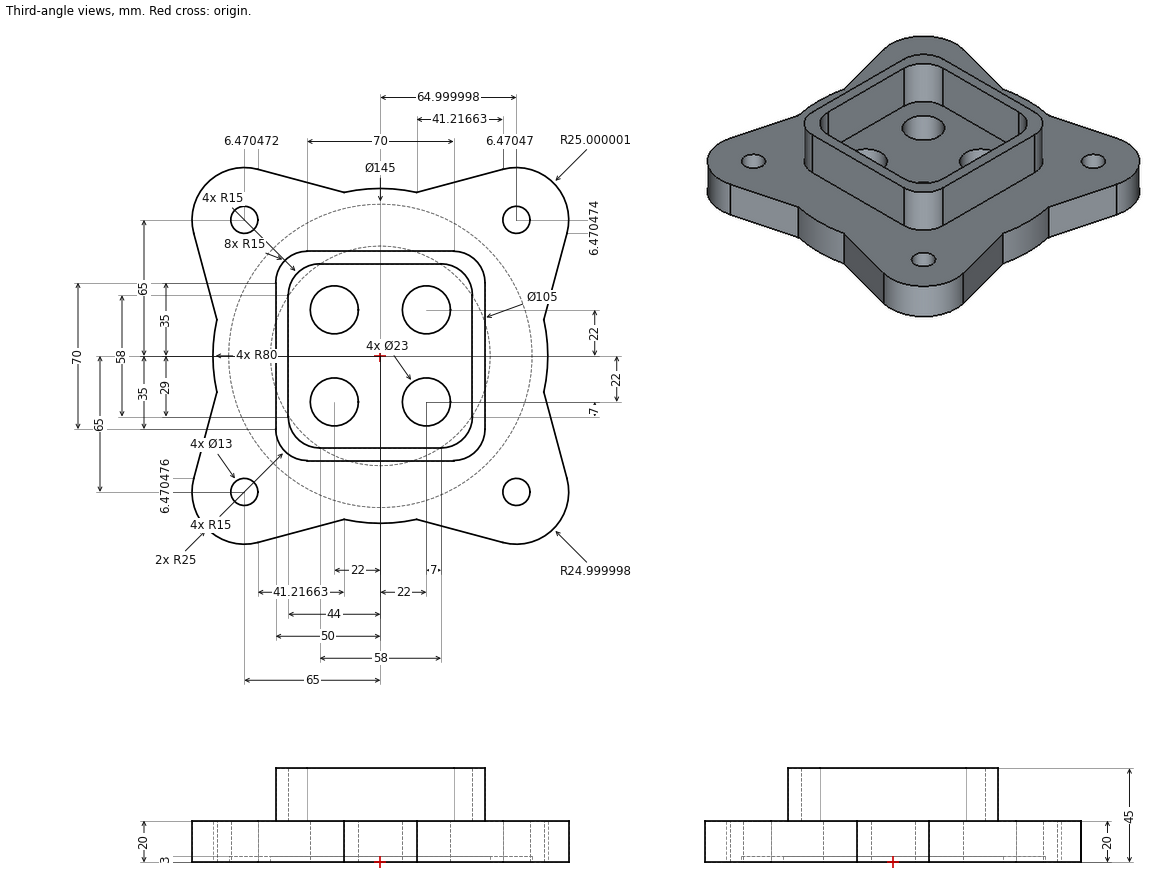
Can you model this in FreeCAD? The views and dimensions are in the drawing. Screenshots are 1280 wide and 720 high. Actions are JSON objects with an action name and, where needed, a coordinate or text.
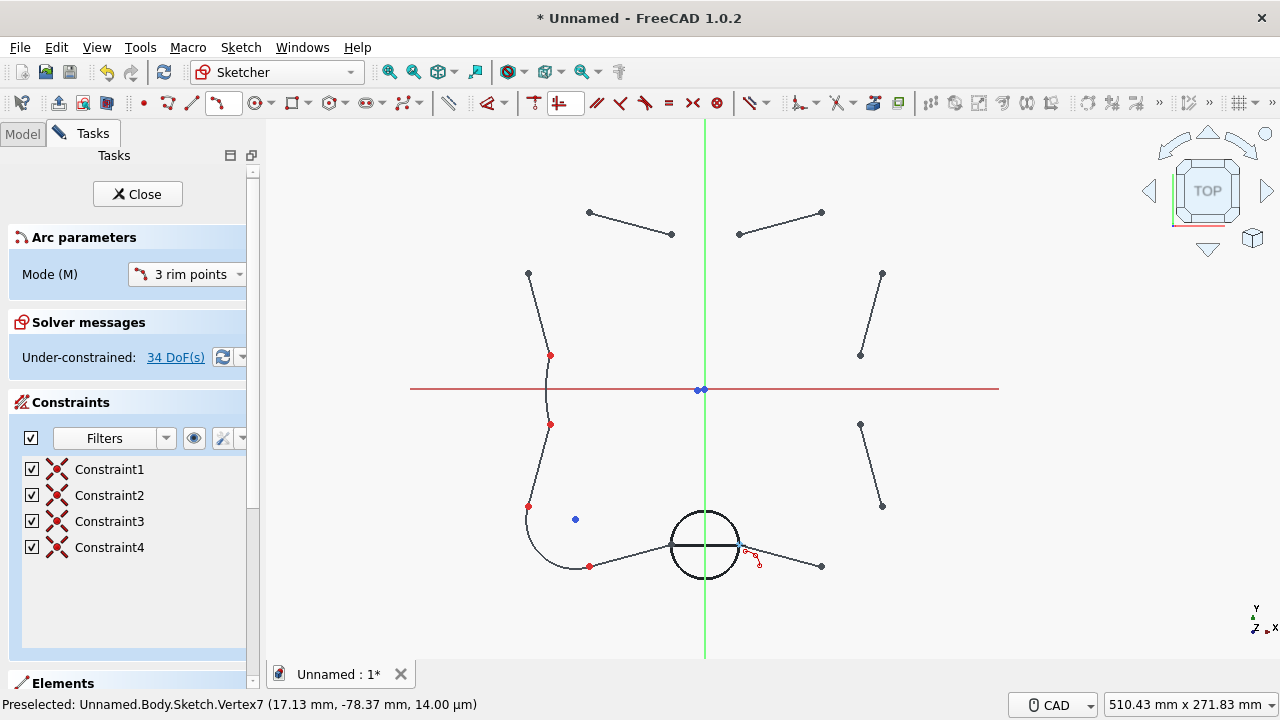
{"action": "scroll", "coordinate": [705, 548], "scroll_direction": "up", "scroll_amount": 8}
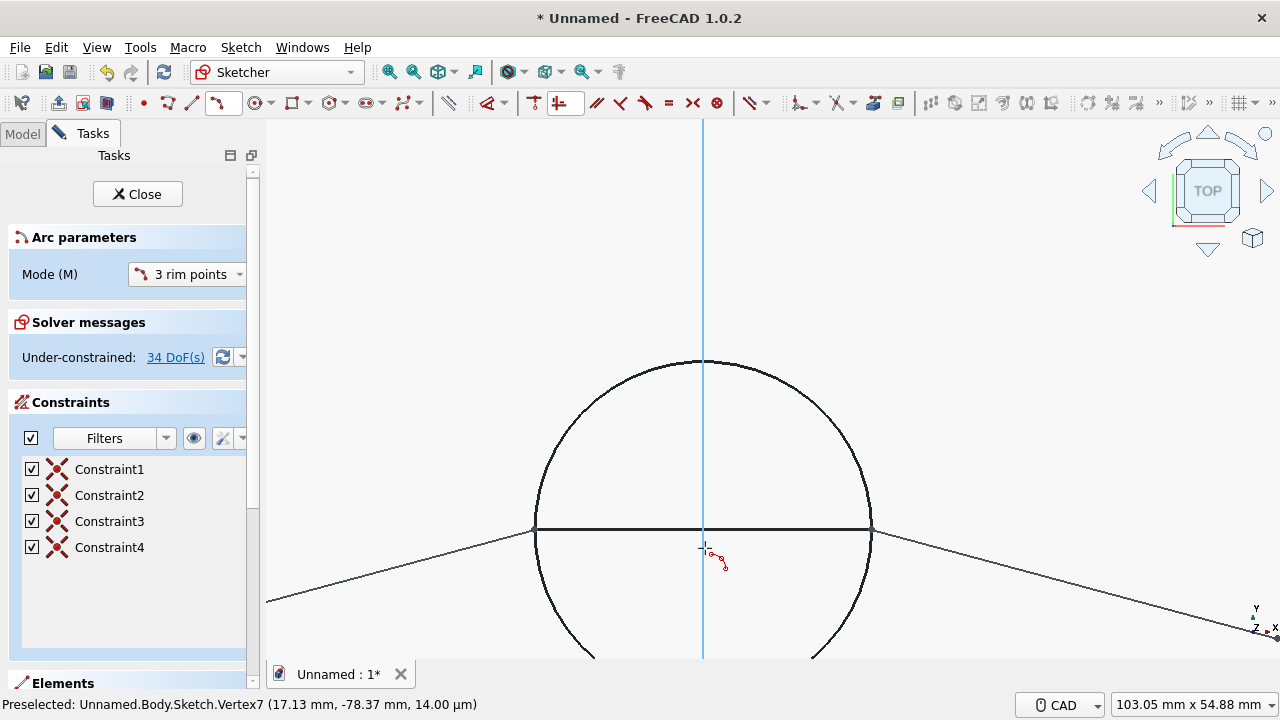
{"action": "left_click", "coordinate": [703, 546]}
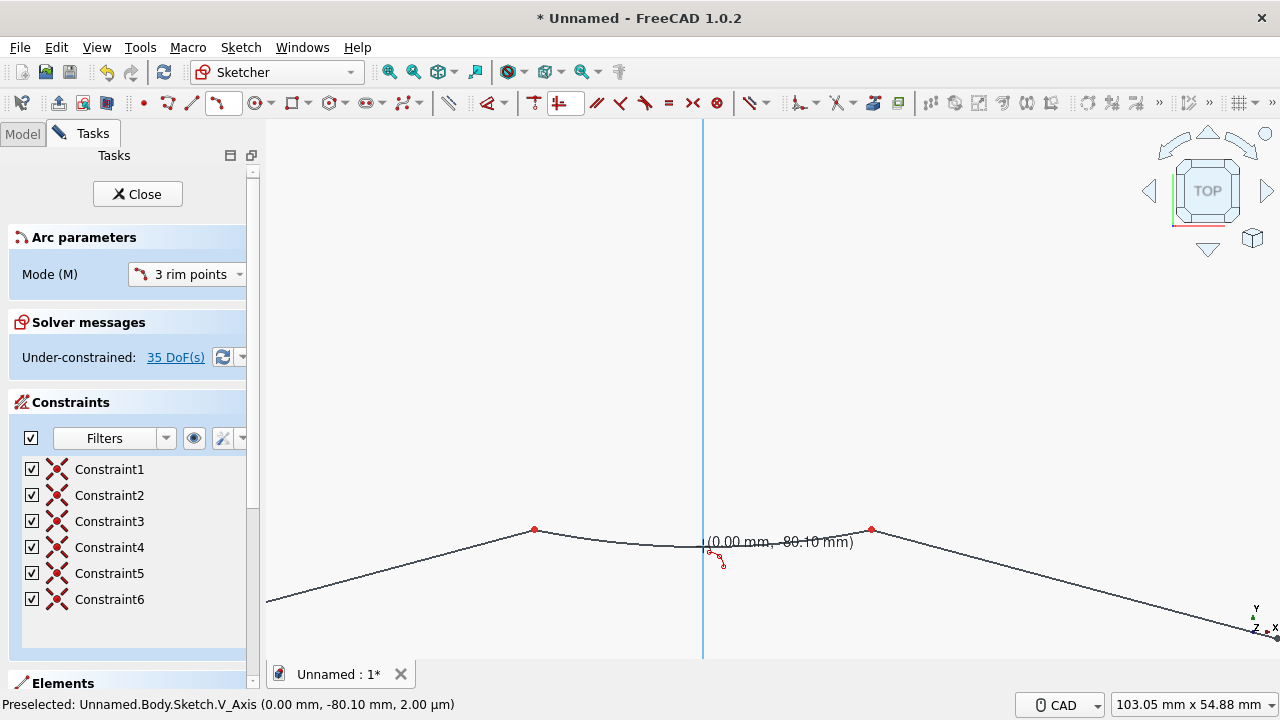
{"action": "scroll", "coordinate": [705, 548], "scroll_direction": "down", "scroll_amount": 8}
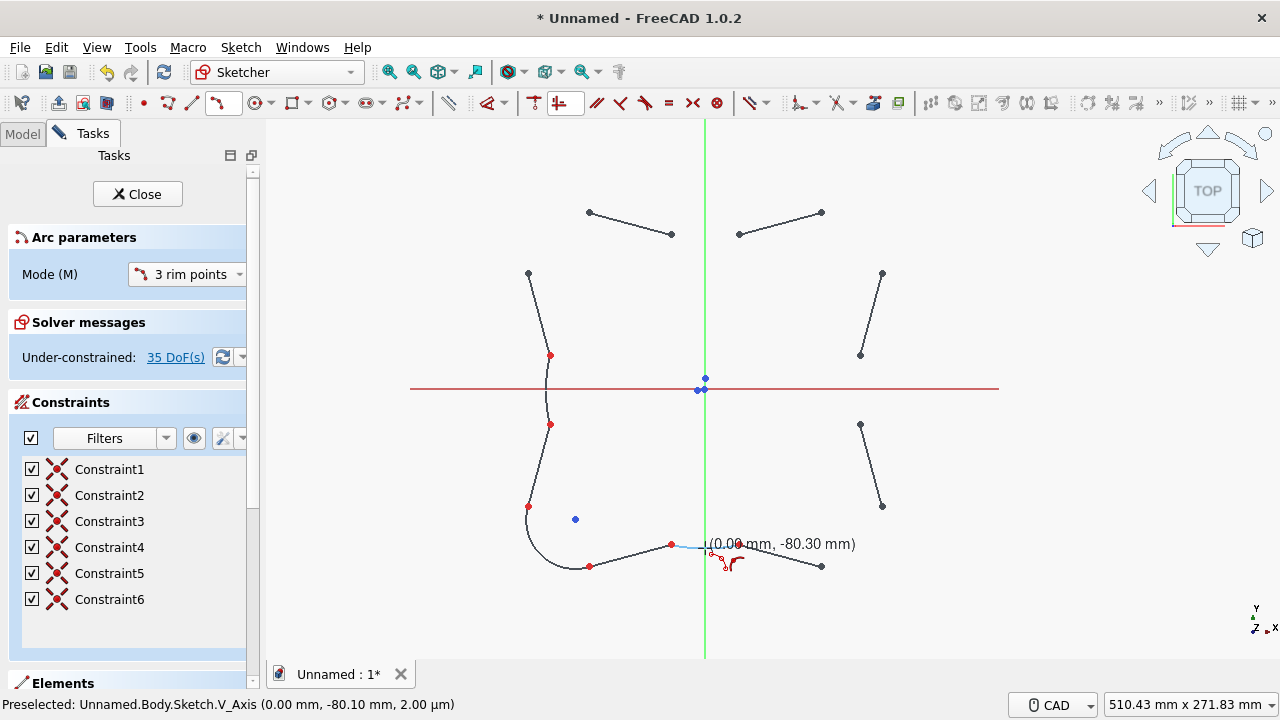
{"action": "left_click", "coordinate": [821, 567]}
{"action": "left_click", "coordinate": [882, 507]}
{"action": "left_click", "coordinate": [869, 554]}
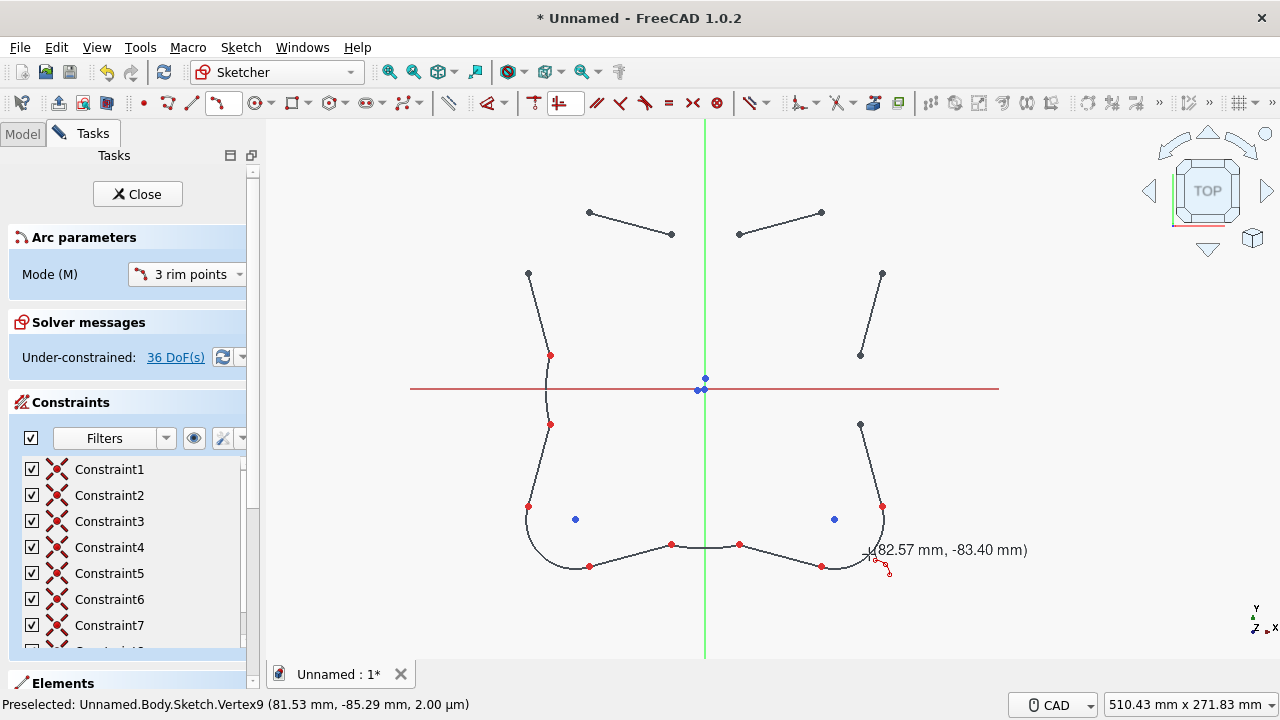
{"action": "left_click", "coordinate": [860, 425]}
{"action": "left_click", "coordinate": [860, 356]}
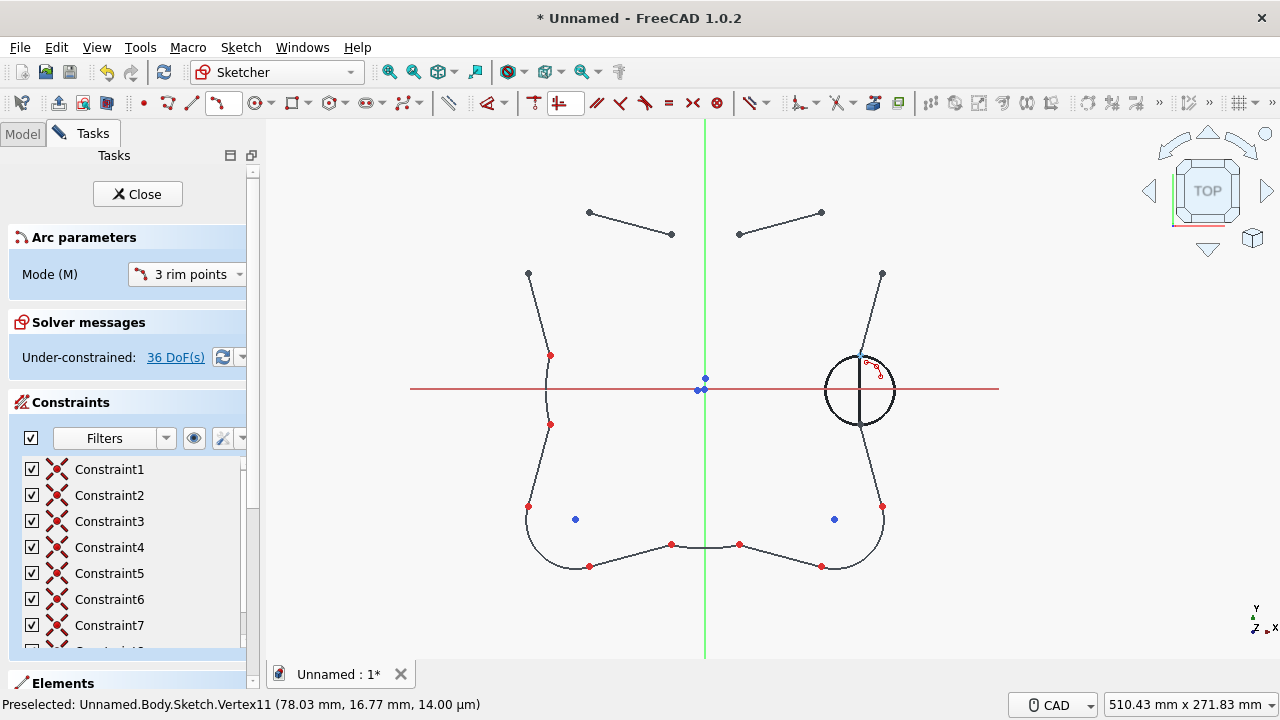
{"action": "scroll", "coordinate": [864, 396], "scroll_direction": "up", "scroll_amount": 8}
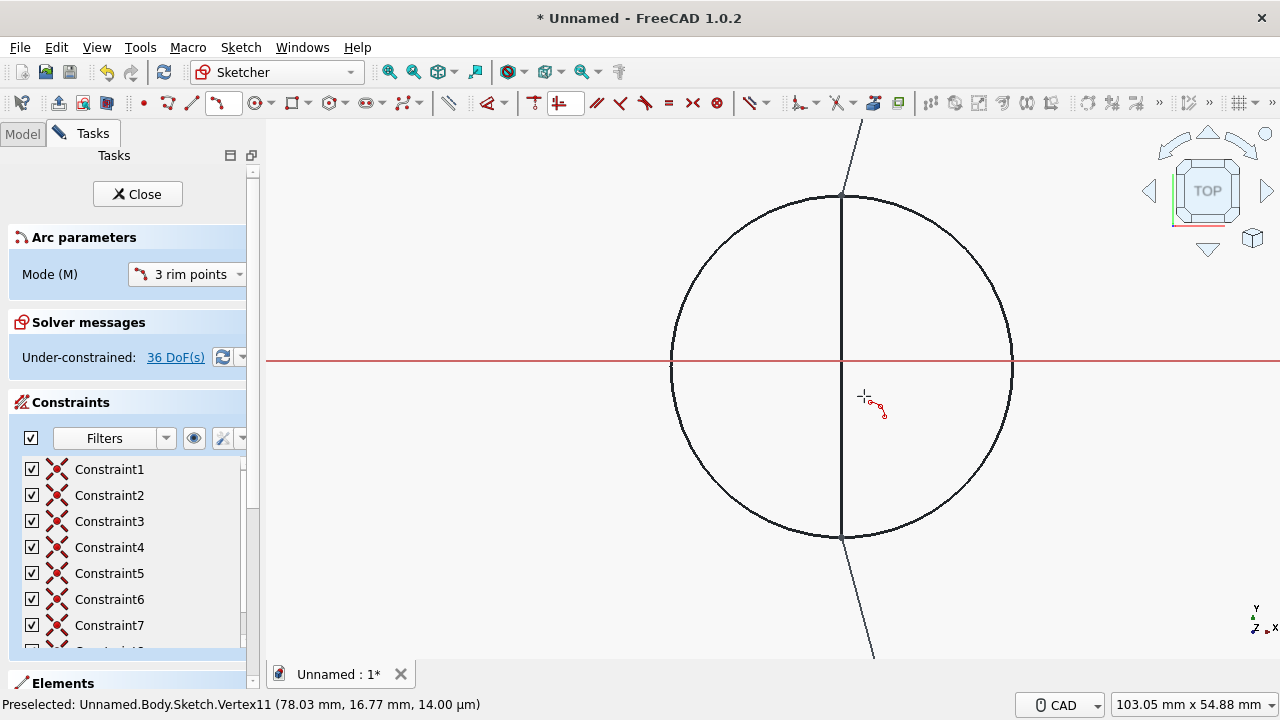
{"action": "left_click", "coordinate": [860, 395]}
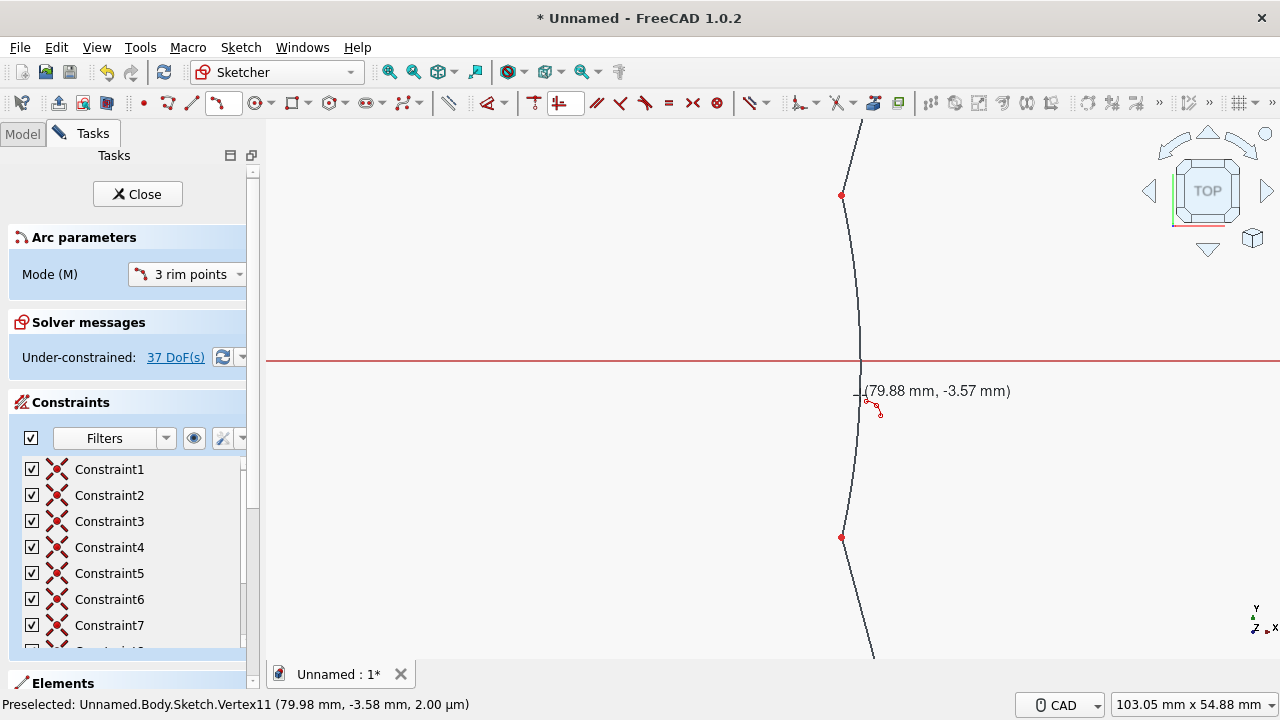
{"action": "scroll", "coordinate": [864, 396], "scroll_direction": "down", "scroll_amount": 8}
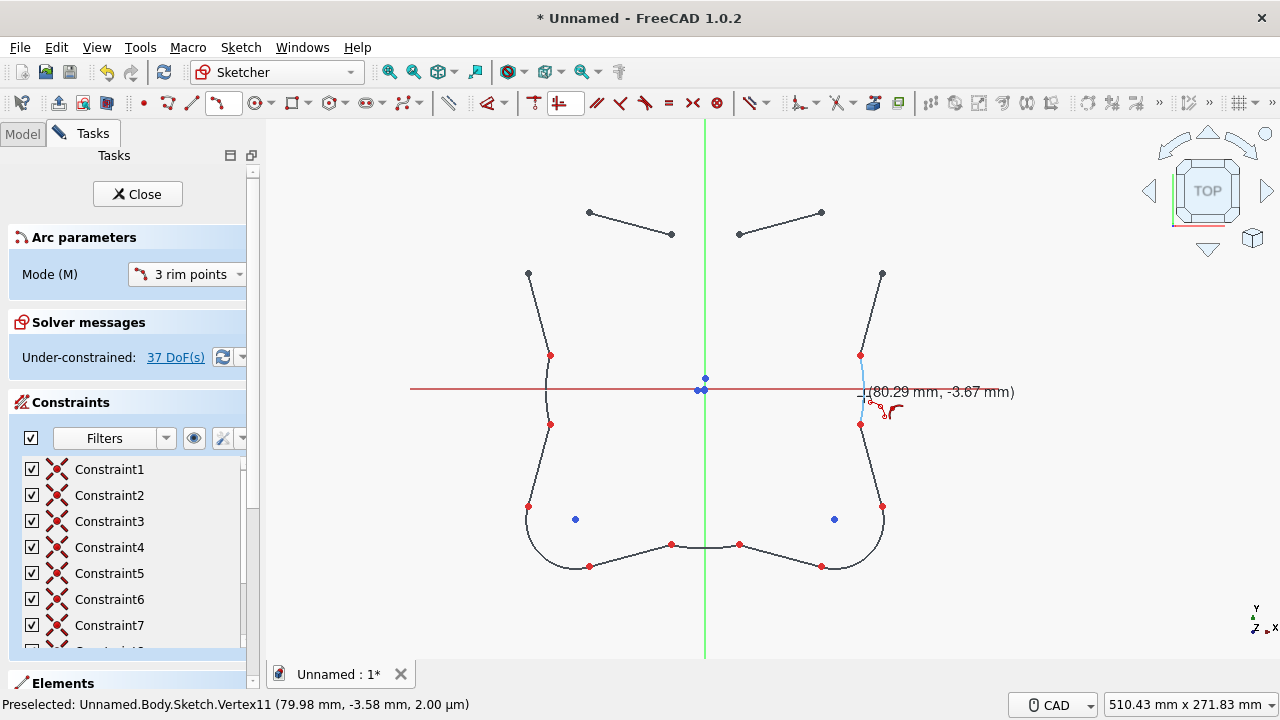
{"action": "left_click", "coordinate": [882, 274]}
{"action": "left_click", "coordinate": [821, 213]}
{"action": "left_click", "coordinate": [869, 225]}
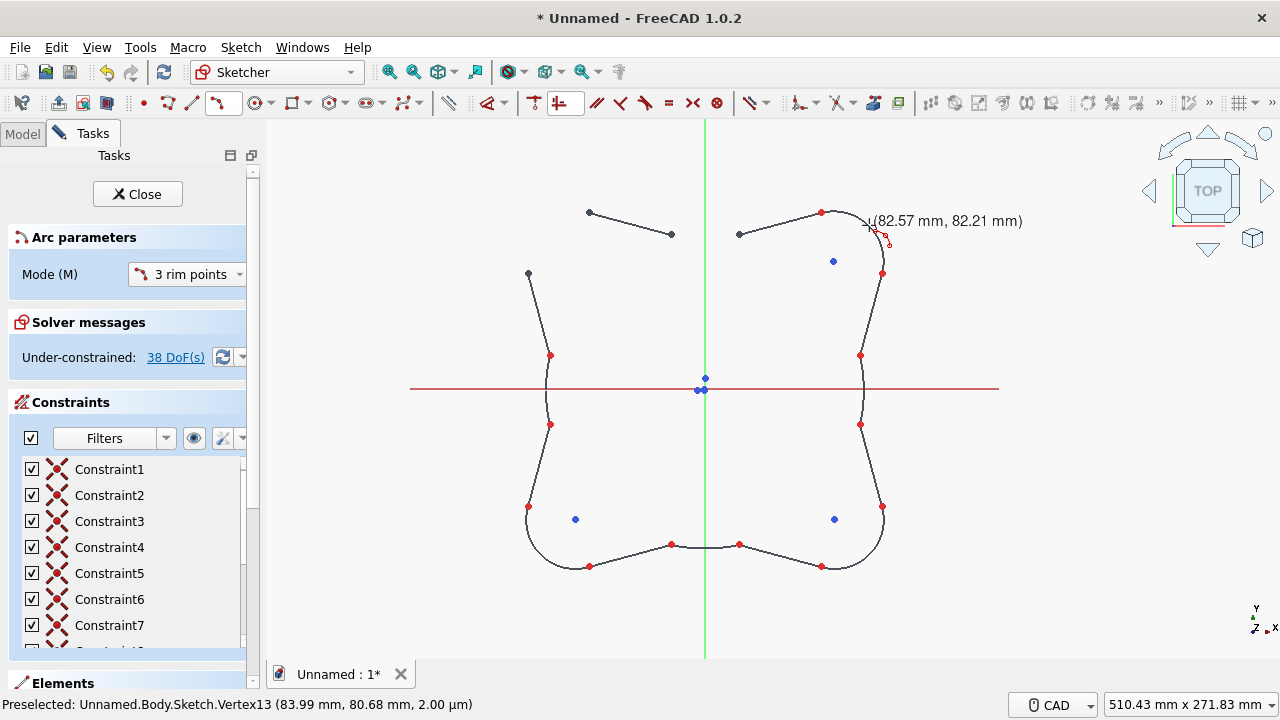
{"action": "left_click", "coordinate": [739, 235]}
{"action": "left_click", "coordinate": [671, 235]}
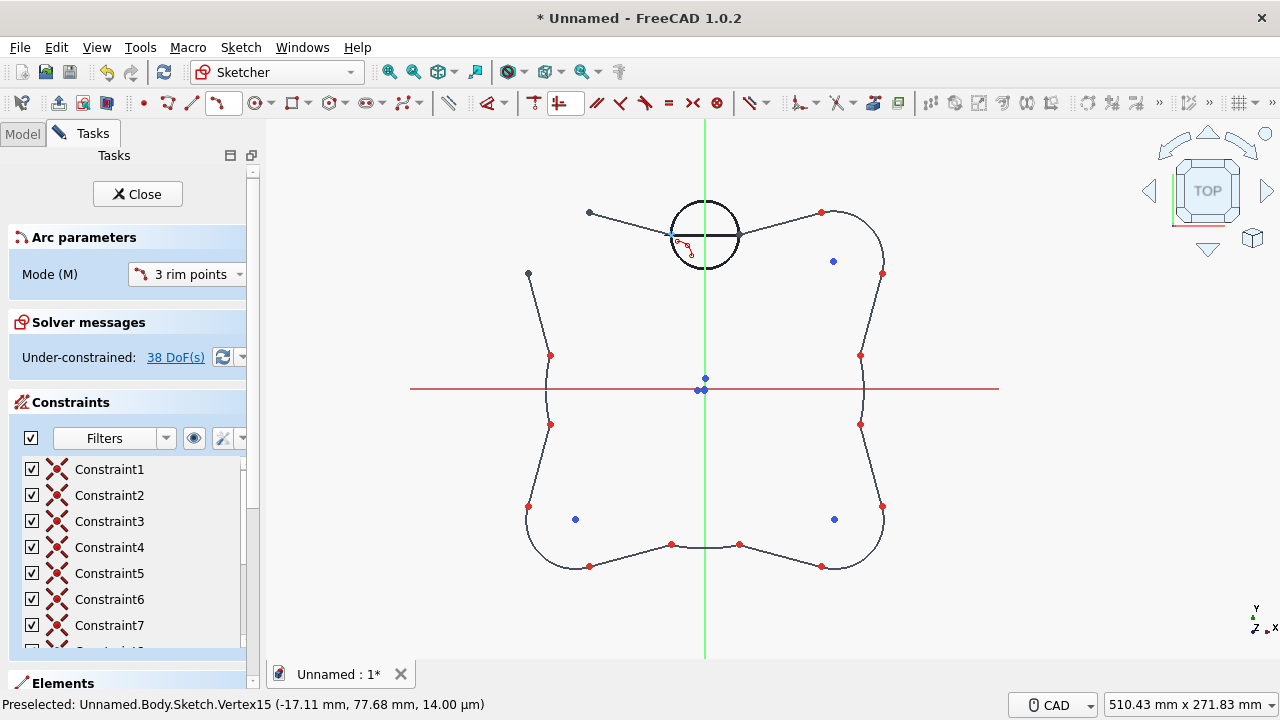
{"action": "scroll", "coordinate": [705, 230], "scroll_direction": "up", "scroll_amount": 8}